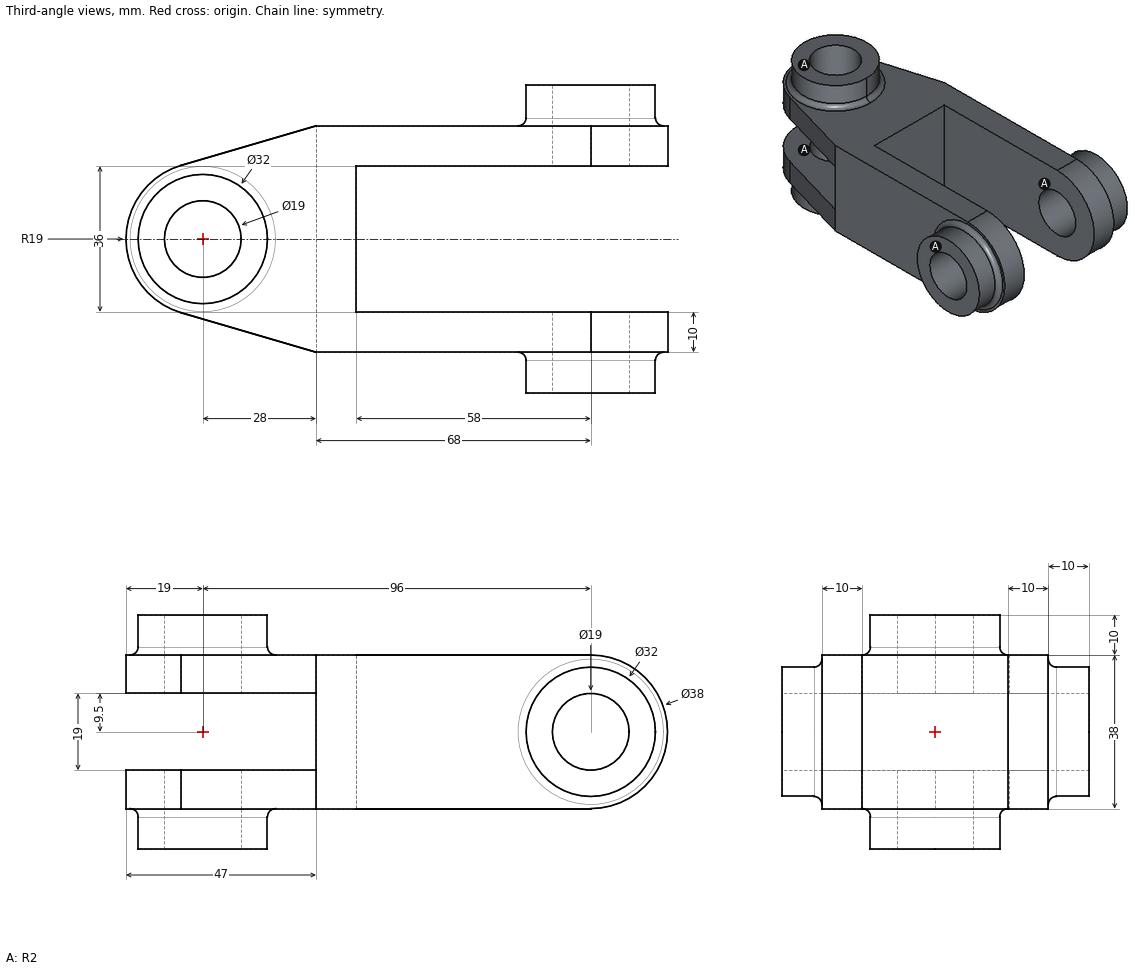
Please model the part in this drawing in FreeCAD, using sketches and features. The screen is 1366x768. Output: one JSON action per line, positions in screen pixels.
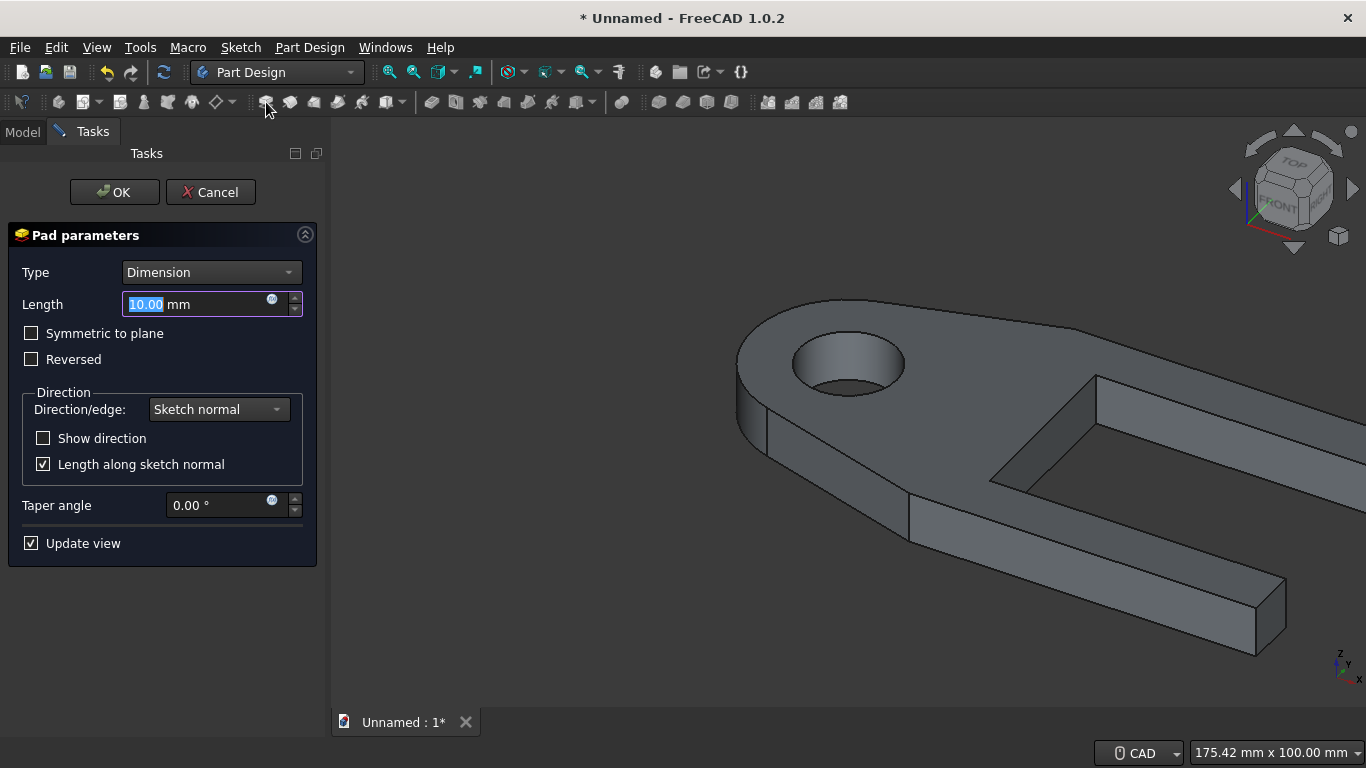
{"action": "type", "text": "38"}
{"action": "key", "text": "Tab"}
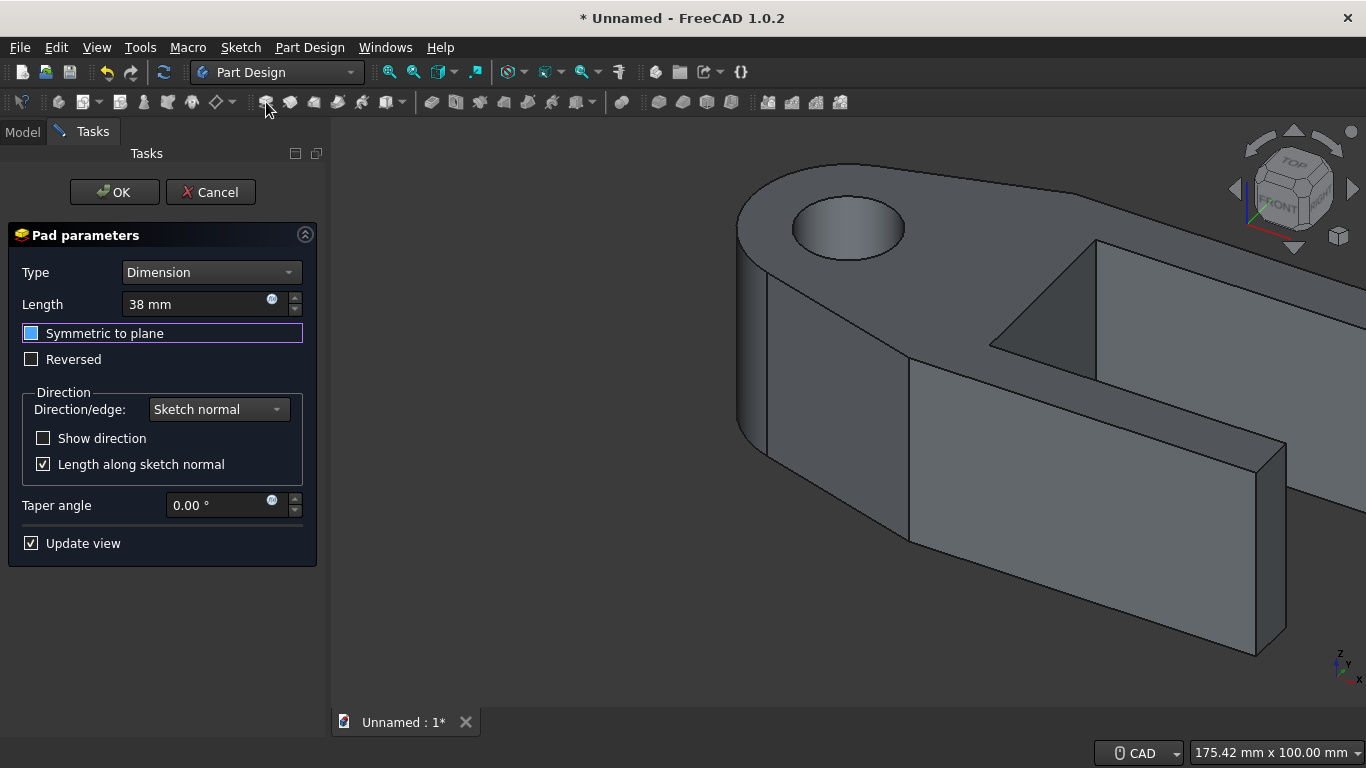
{"action": "left_click", "coordinate": [30, 333]}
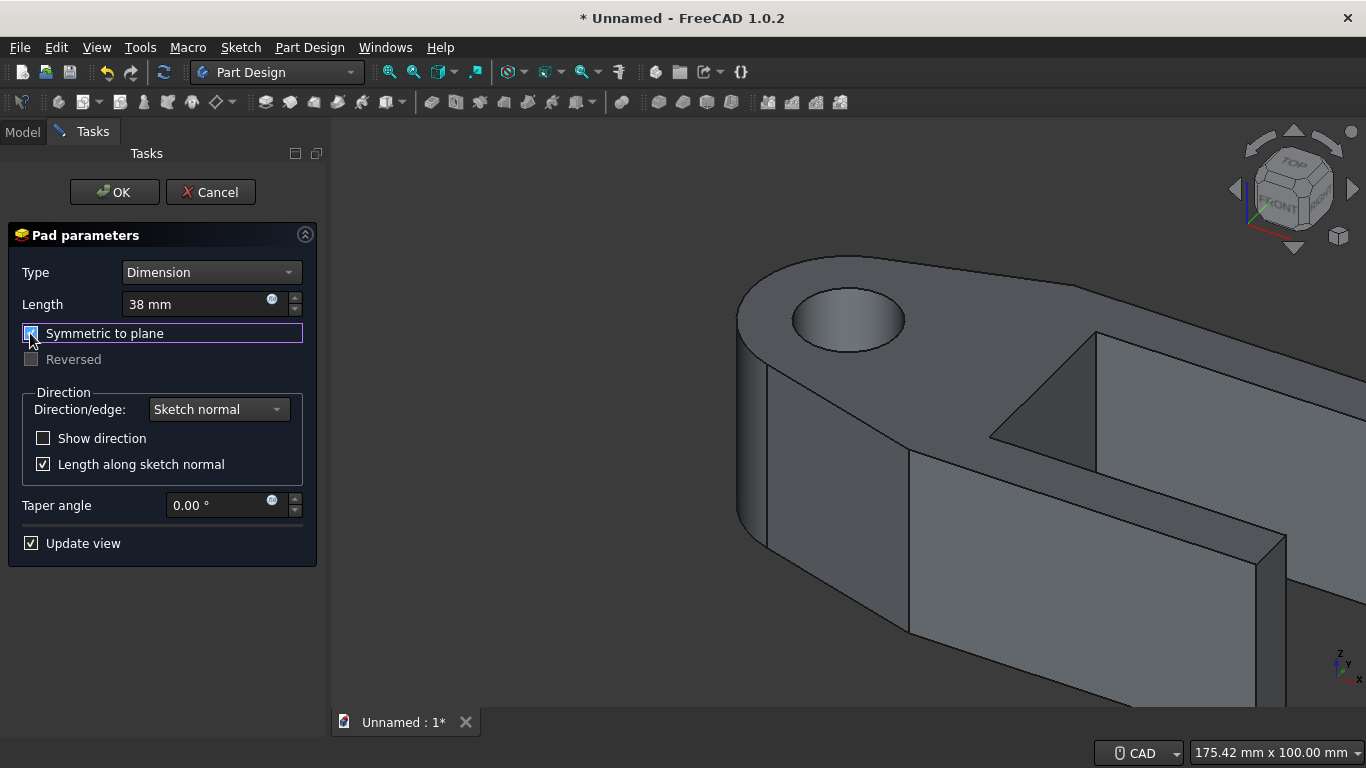
{"action": "left_click", "coordinate": [115, 192]}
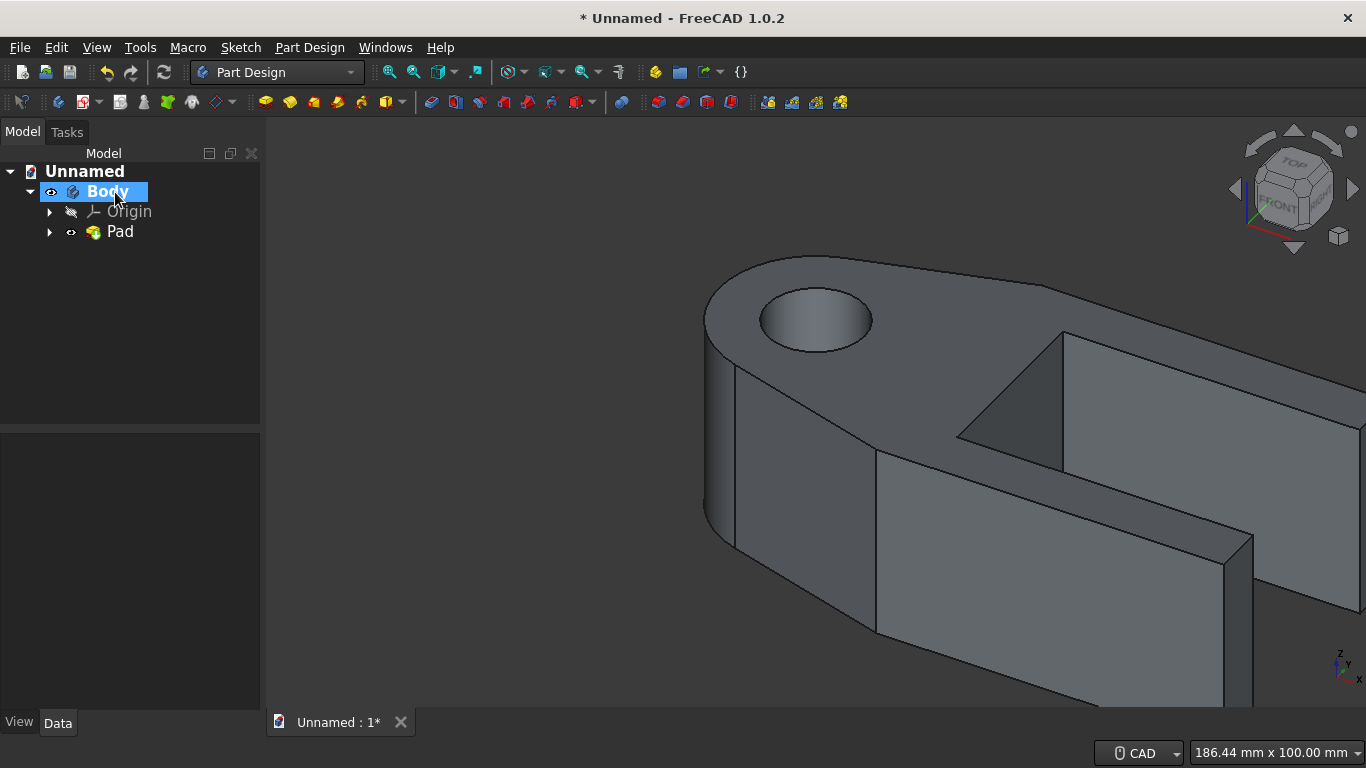
{"action": "left_click", "coordinate": [390, 72]}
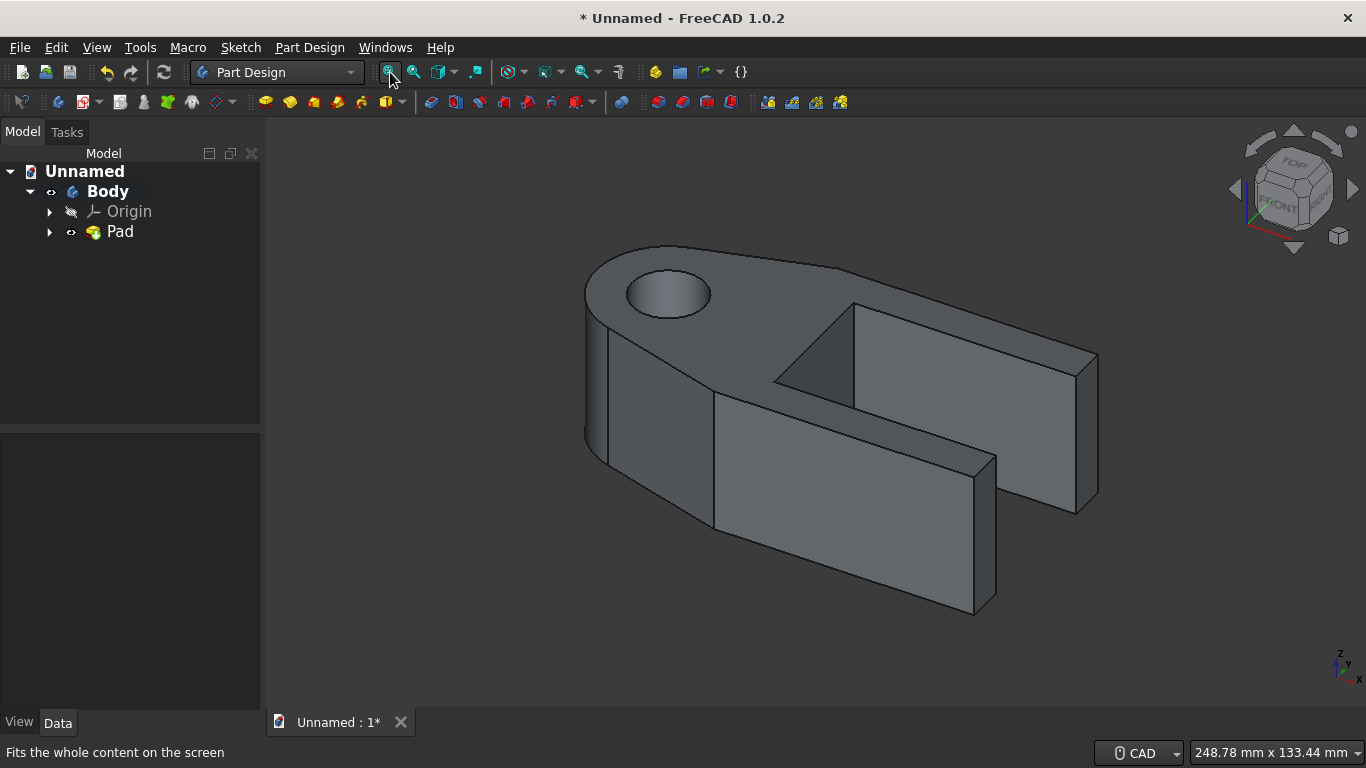
{"action": "key", "text": "4"}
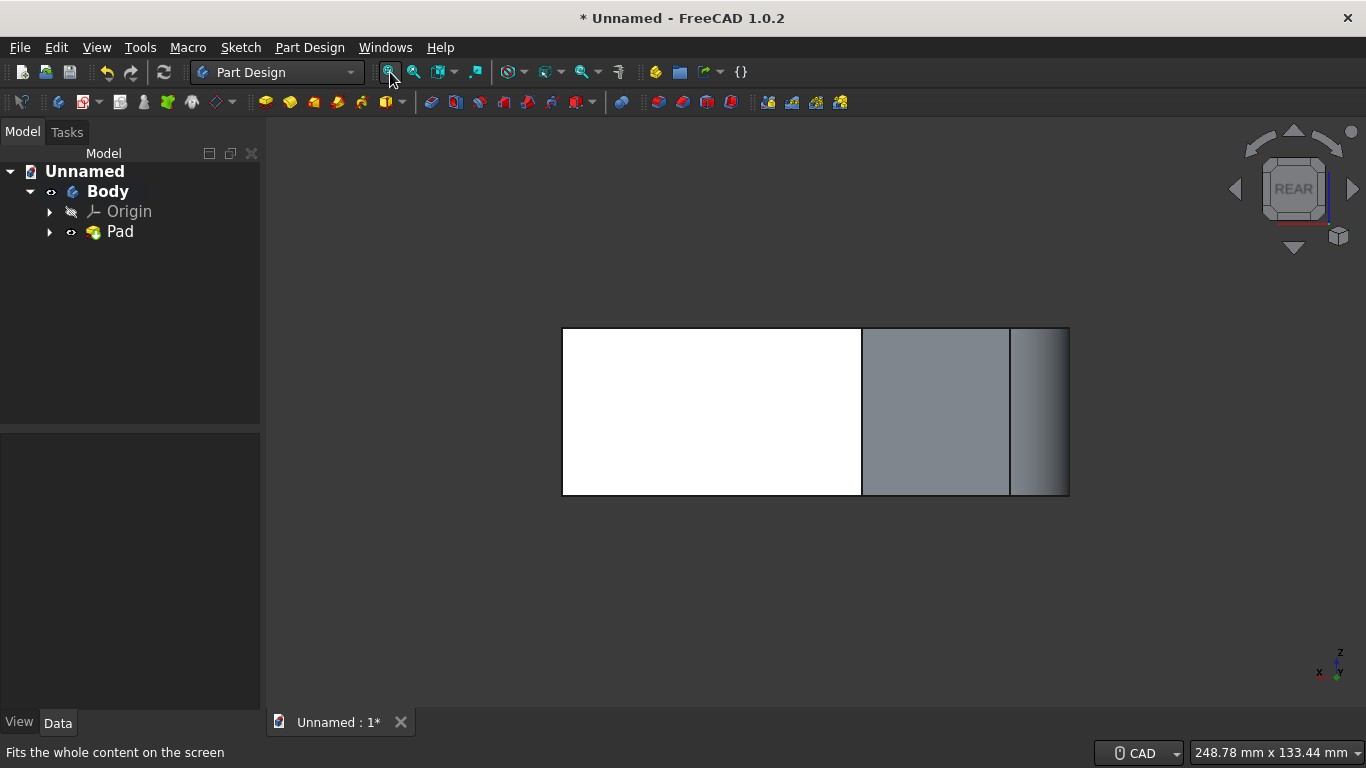
{"action": "left_click", "coordinate": [669, 411]}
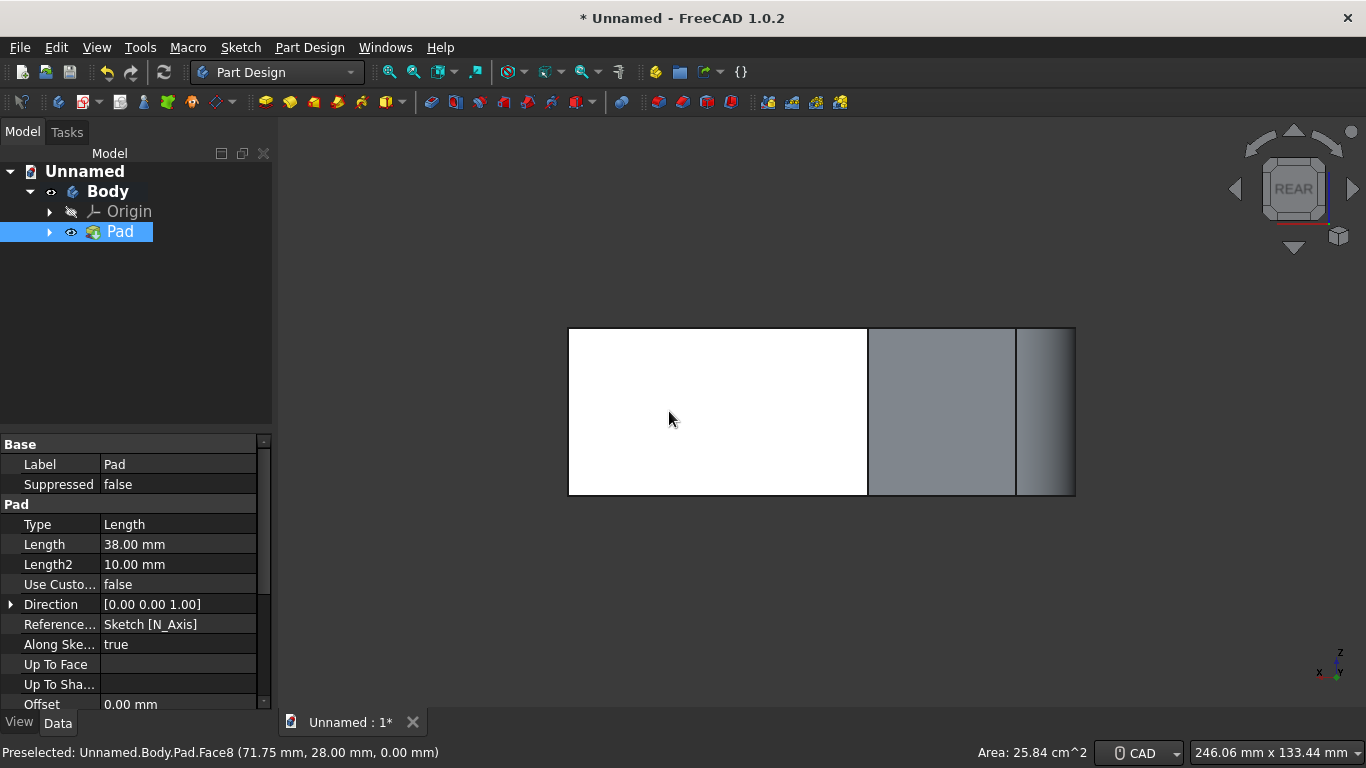
{"action": "left_click", "coordinate": [84, 102]}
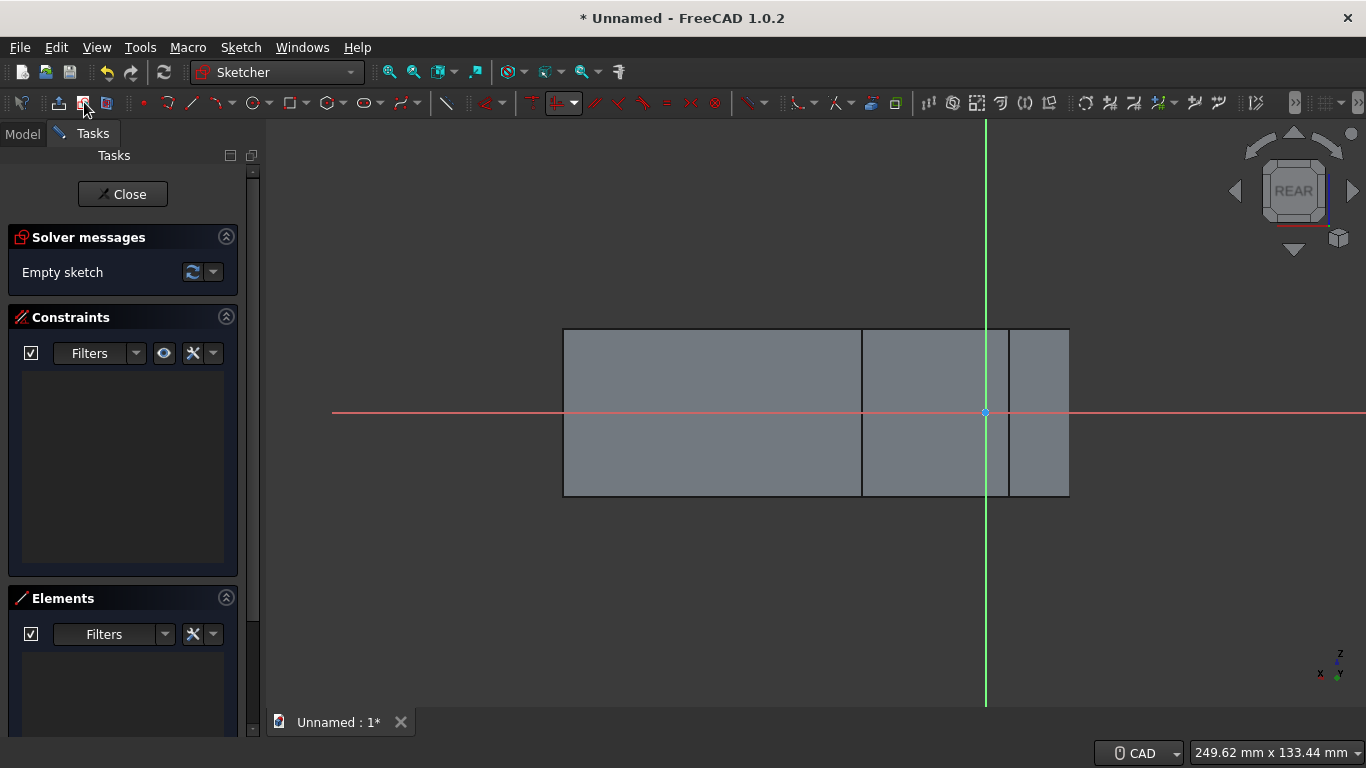
{"action": "scroll", "coordinate": [412, 413], "scroll_direction": "up", "scroll_amount": 4}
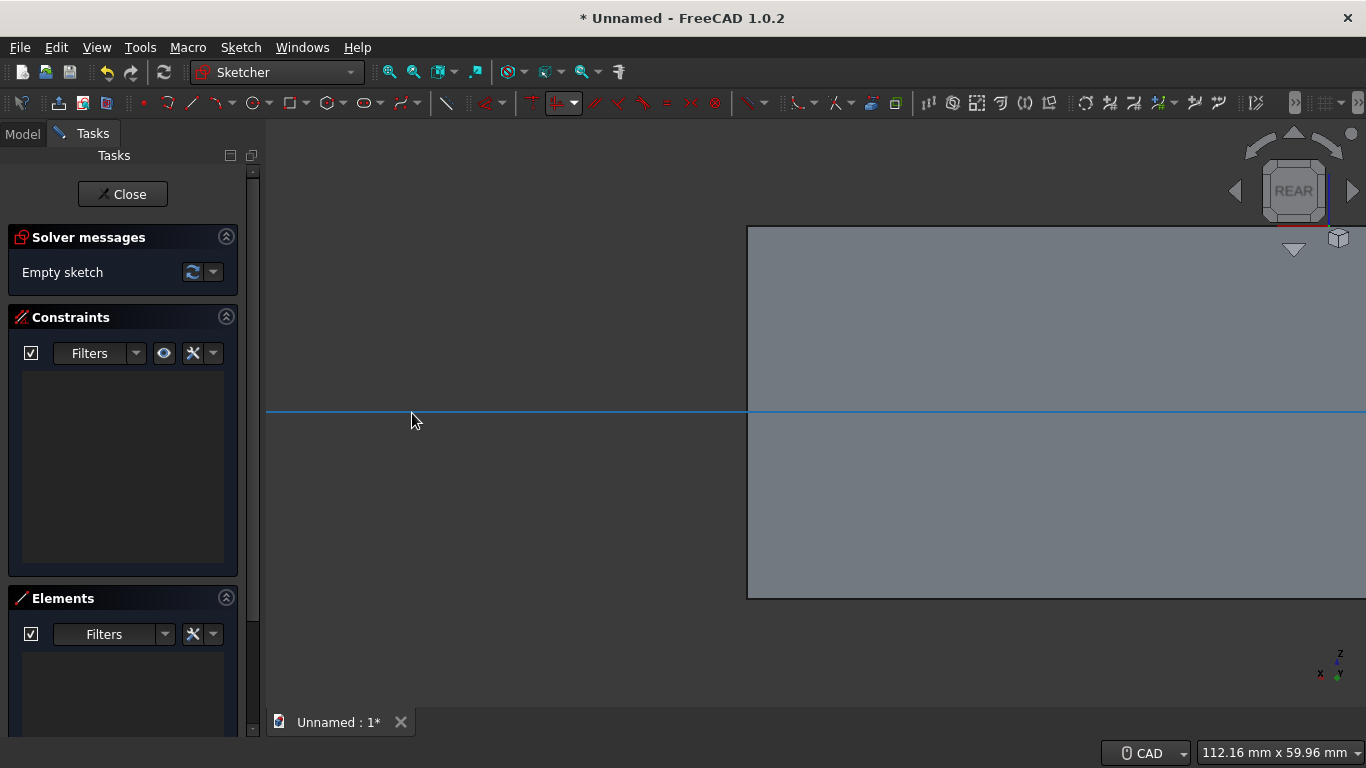
{"action": "left_click", "coordinate": [254, 104]}